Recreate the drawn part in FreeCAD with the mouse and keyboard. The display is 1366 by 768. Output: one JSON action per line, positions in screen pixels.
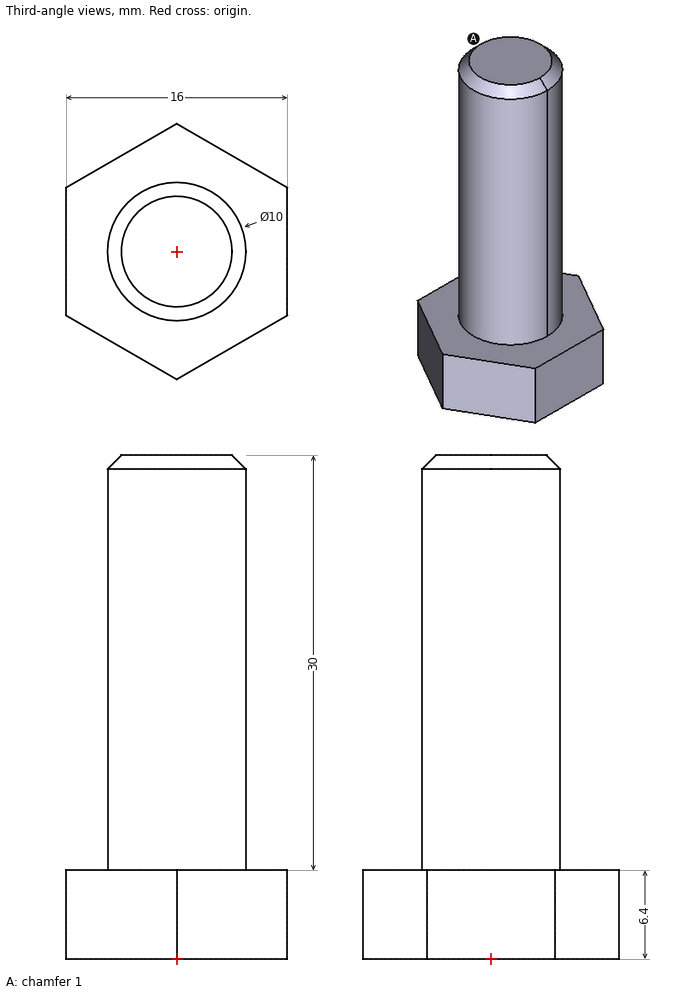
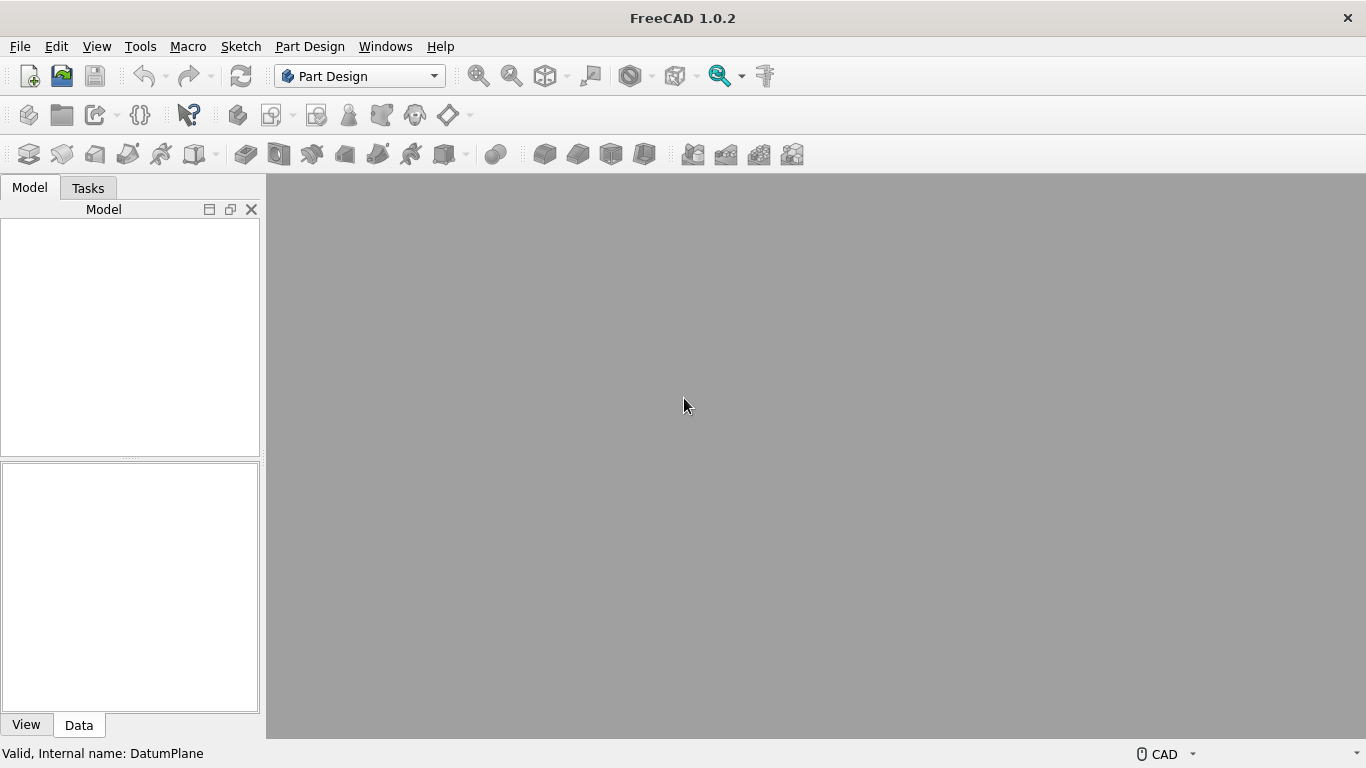
{"action": "left_click", "coordinate": [29, 76]}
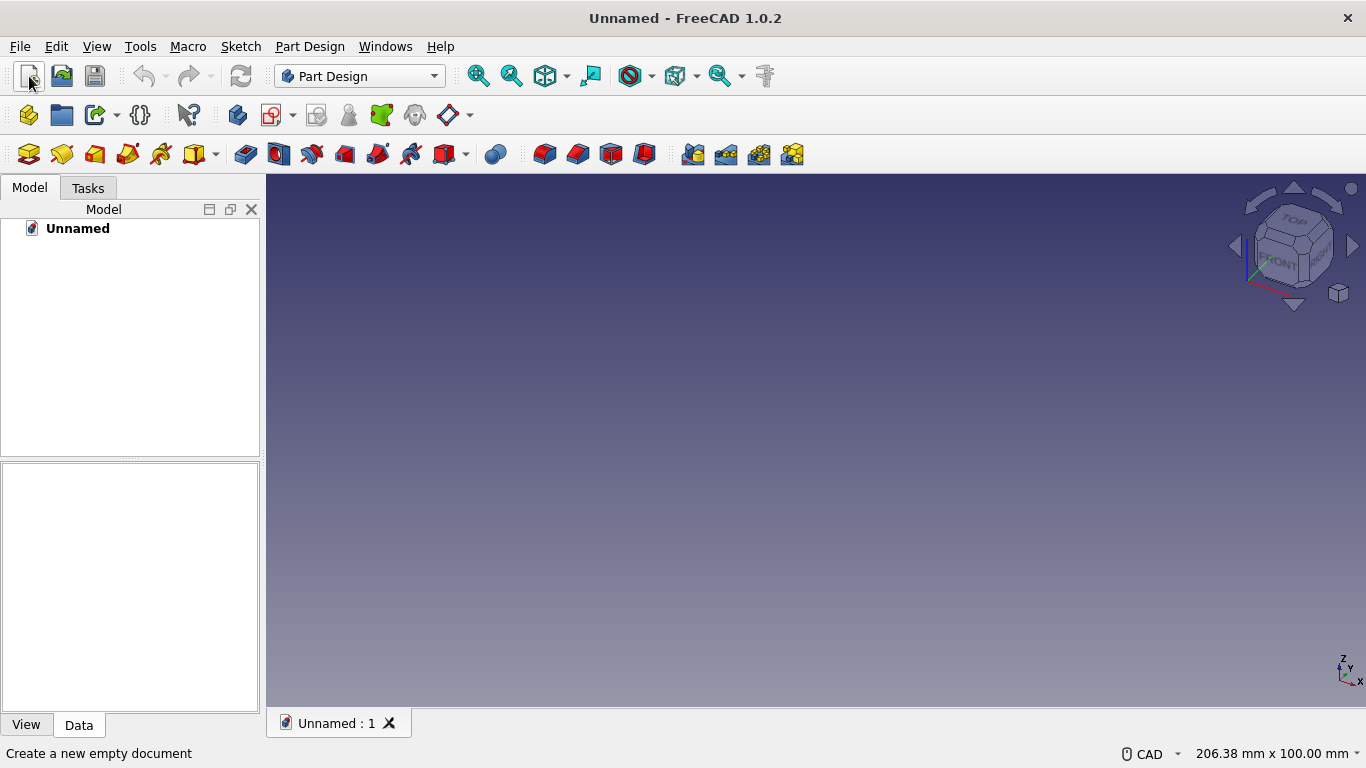
{"action": "left_click", "coordinate": [270, 116]}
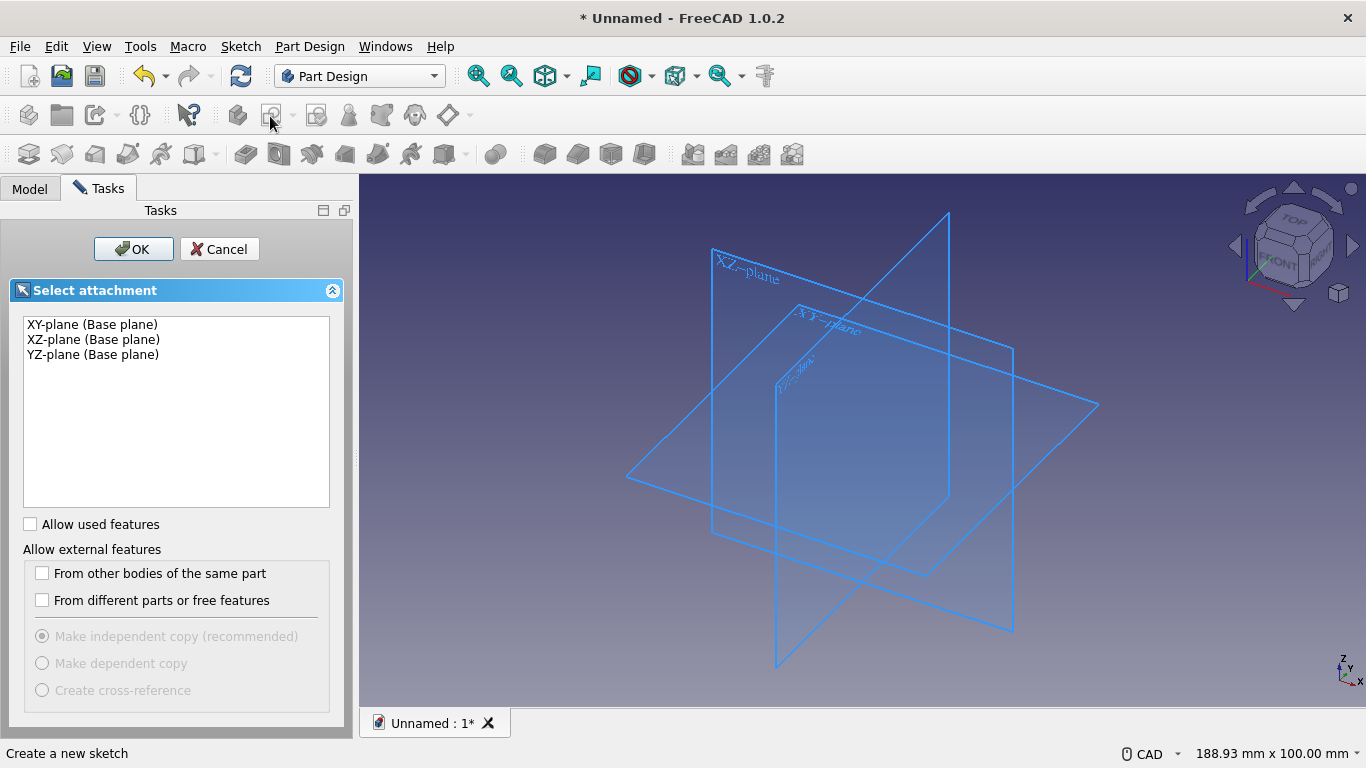
{"action": "left_click", "coordinate": [84, 324]}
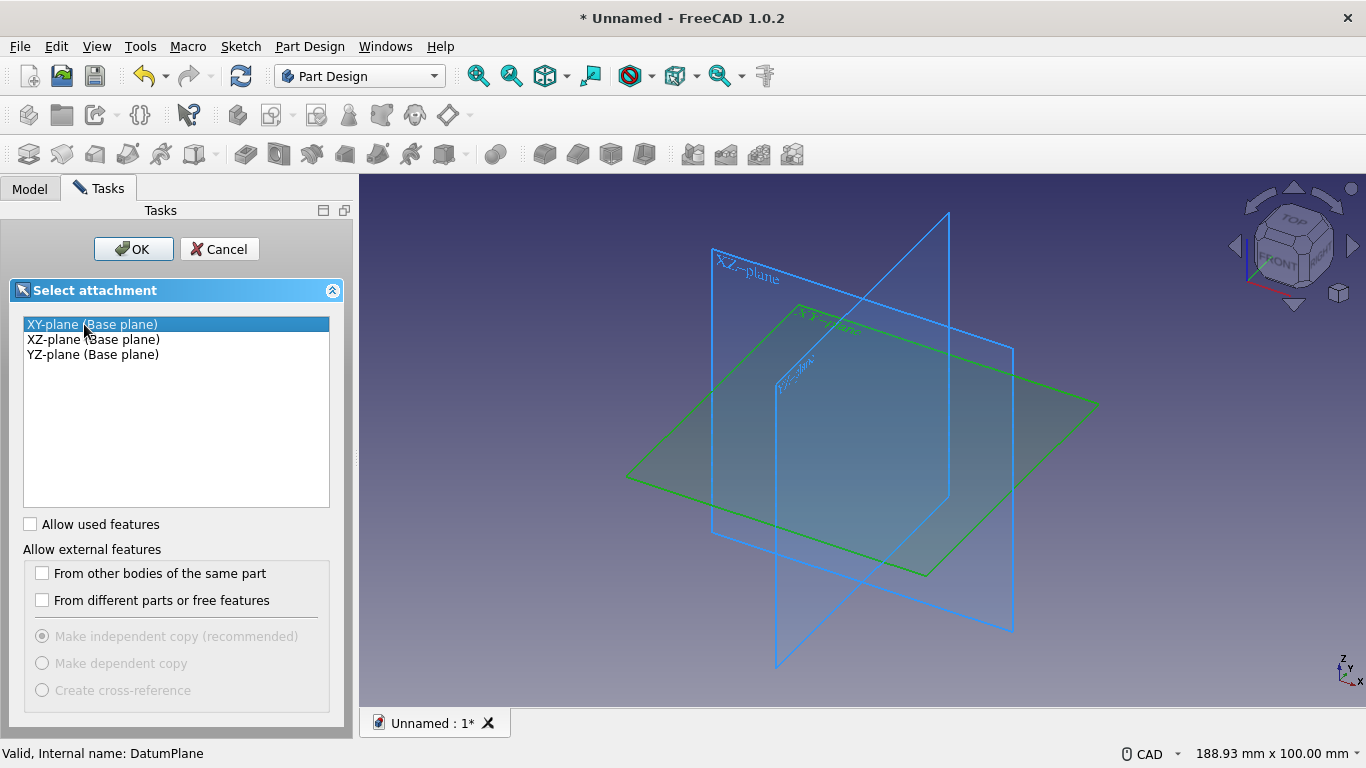
{"action": "left_click", "coordinate": [134, 249]}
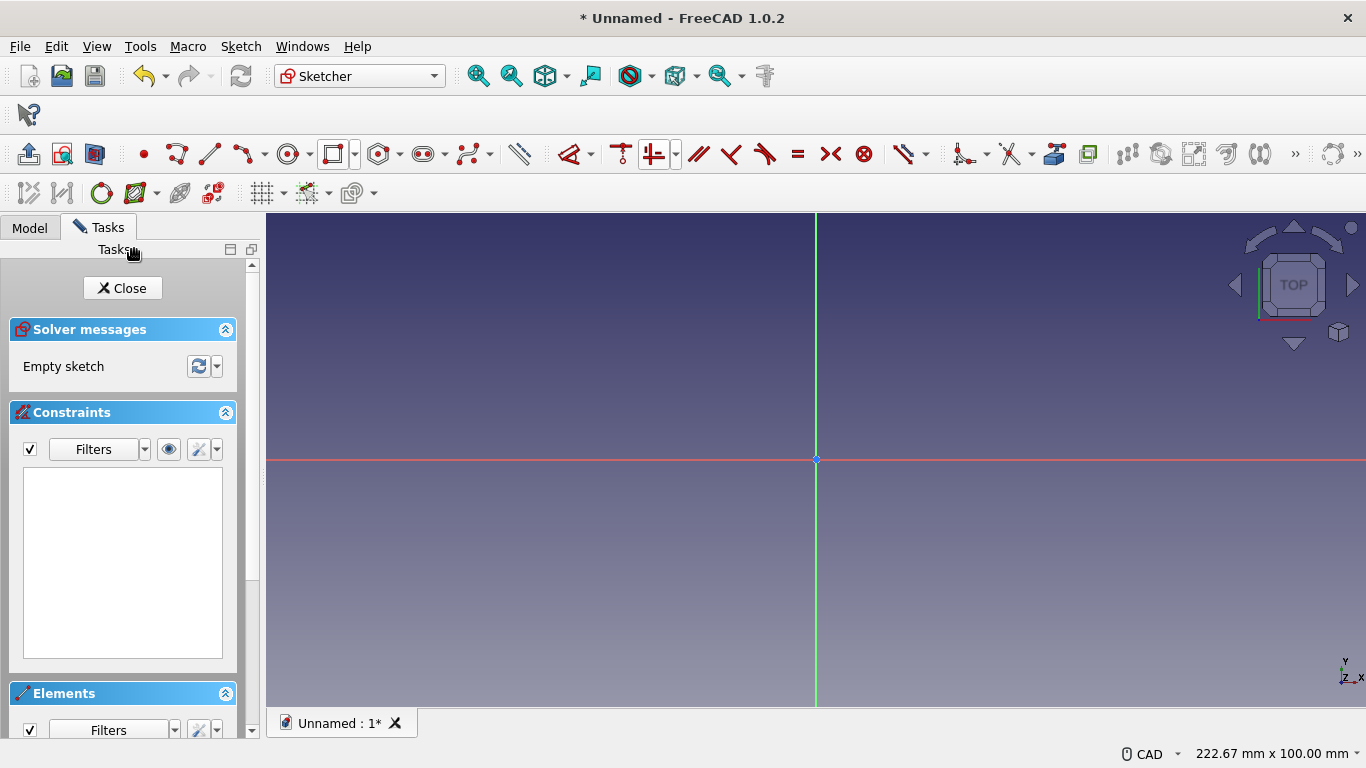
{"action": "scroll", "coordinate": [846, 460], "scroll_direction": "up", "scroll_amount": 6}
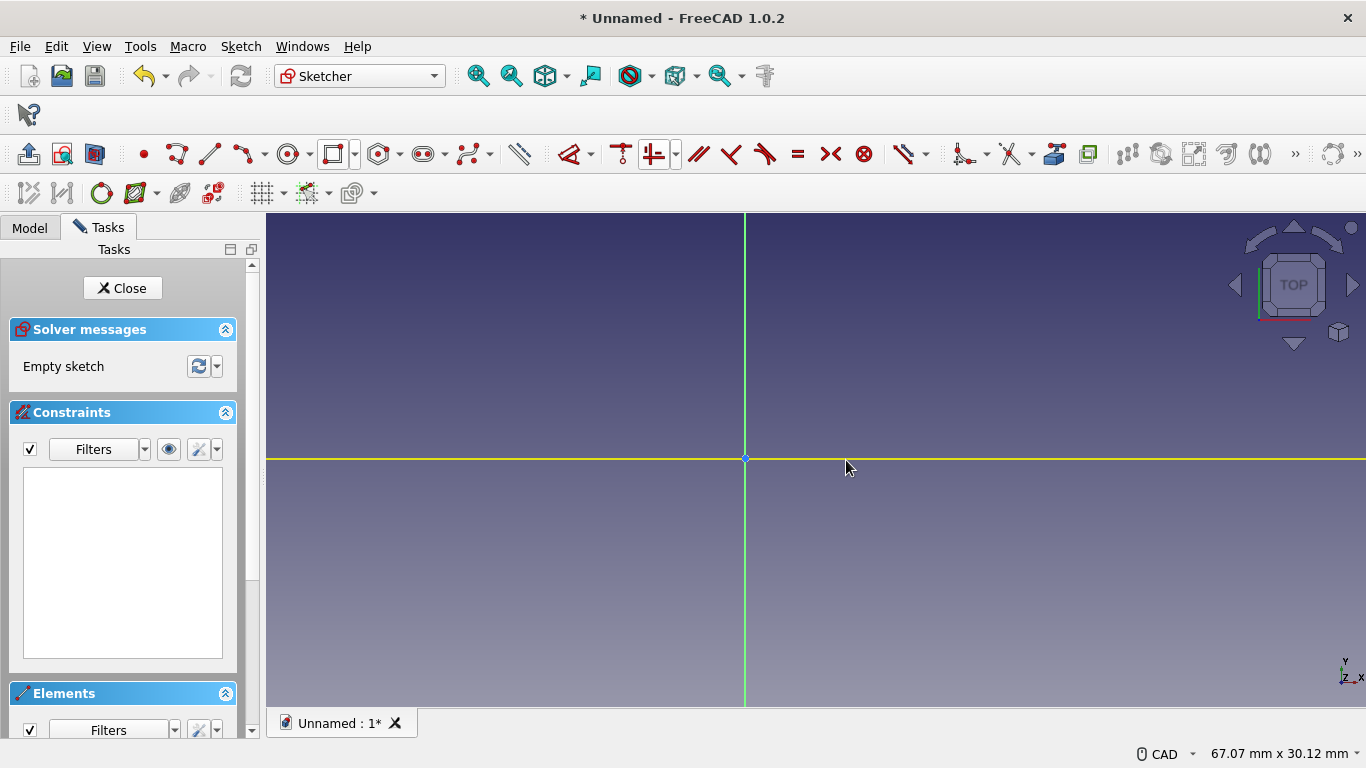
{"action": "key", "text": "g p 6"}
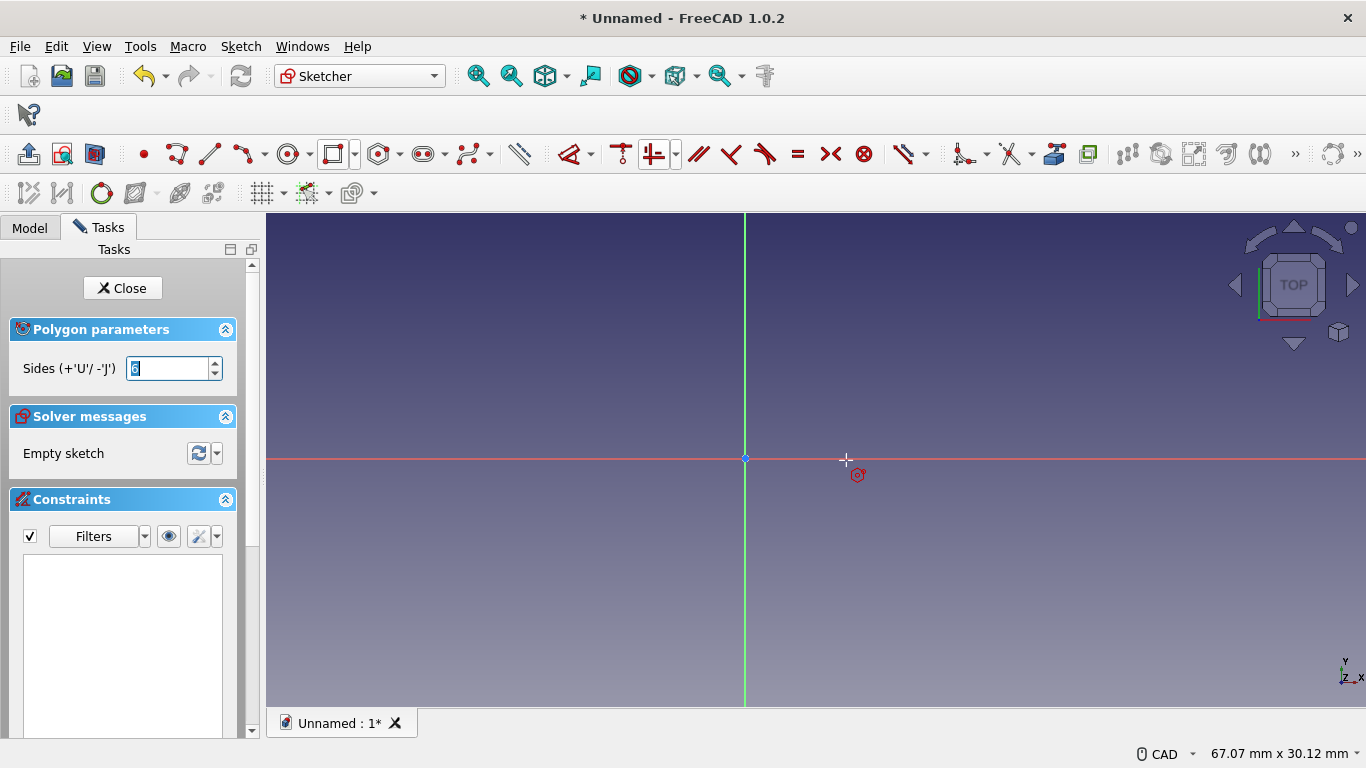
{"action": "left_click", "coordinate": [745, 459]}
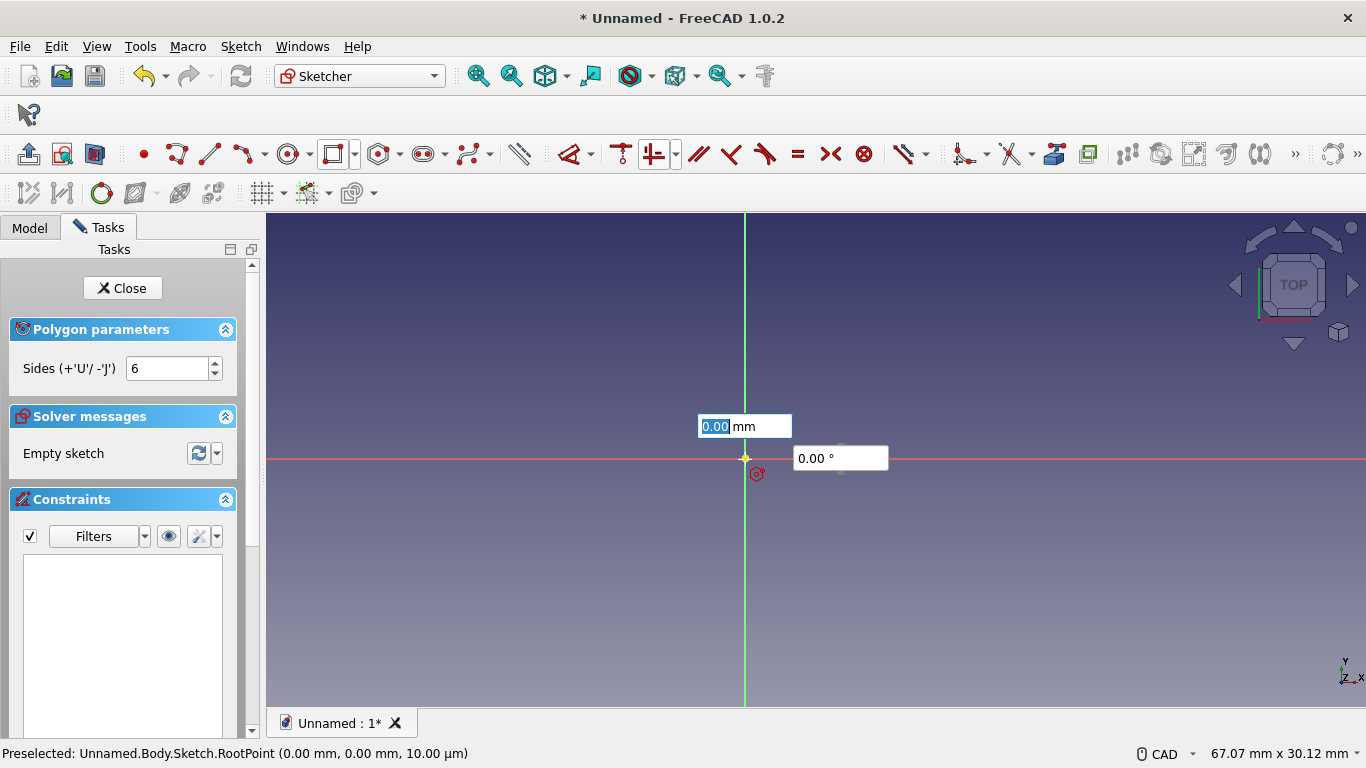
{"action": "left_click", "coordinate": [745, 307]}
{"action": "right_click", "coordinate": [745, 307]}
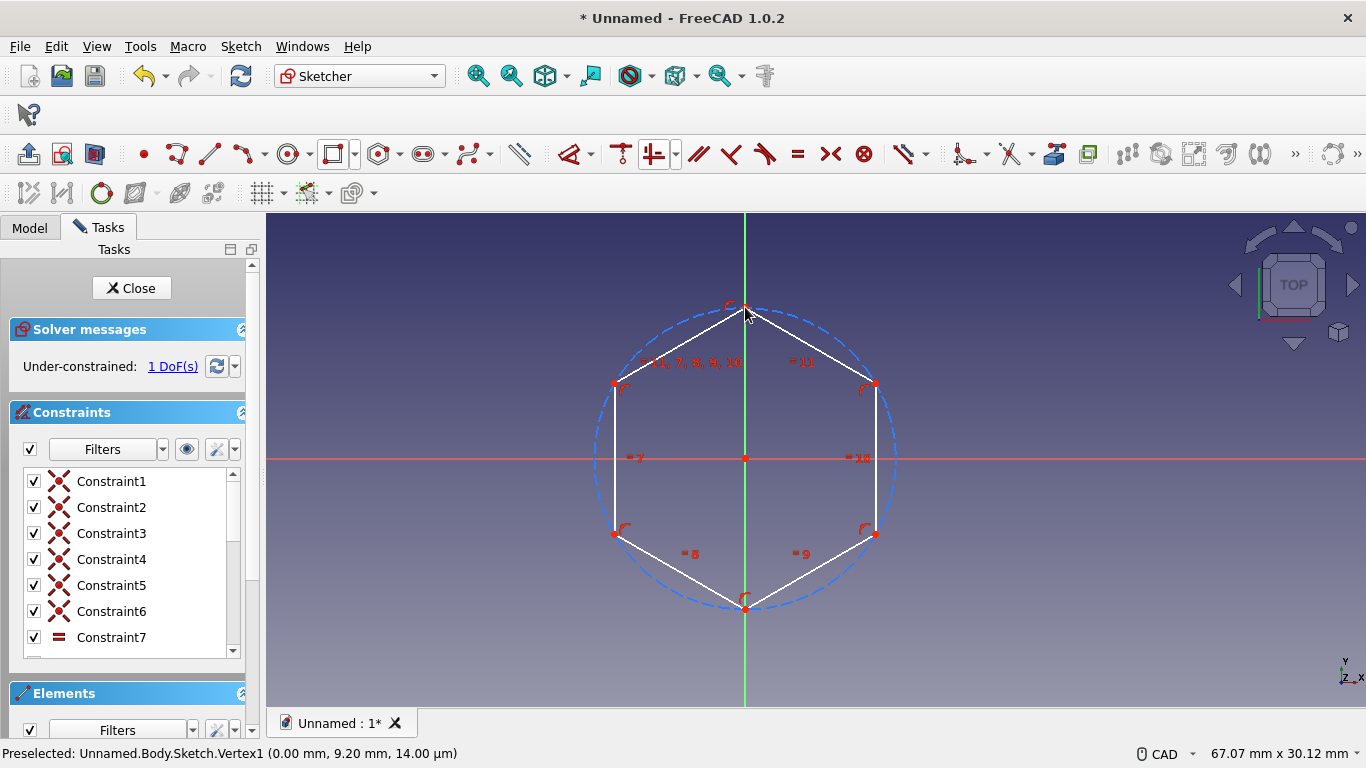
{"action": "left_click", "coordinate": [568, 154]}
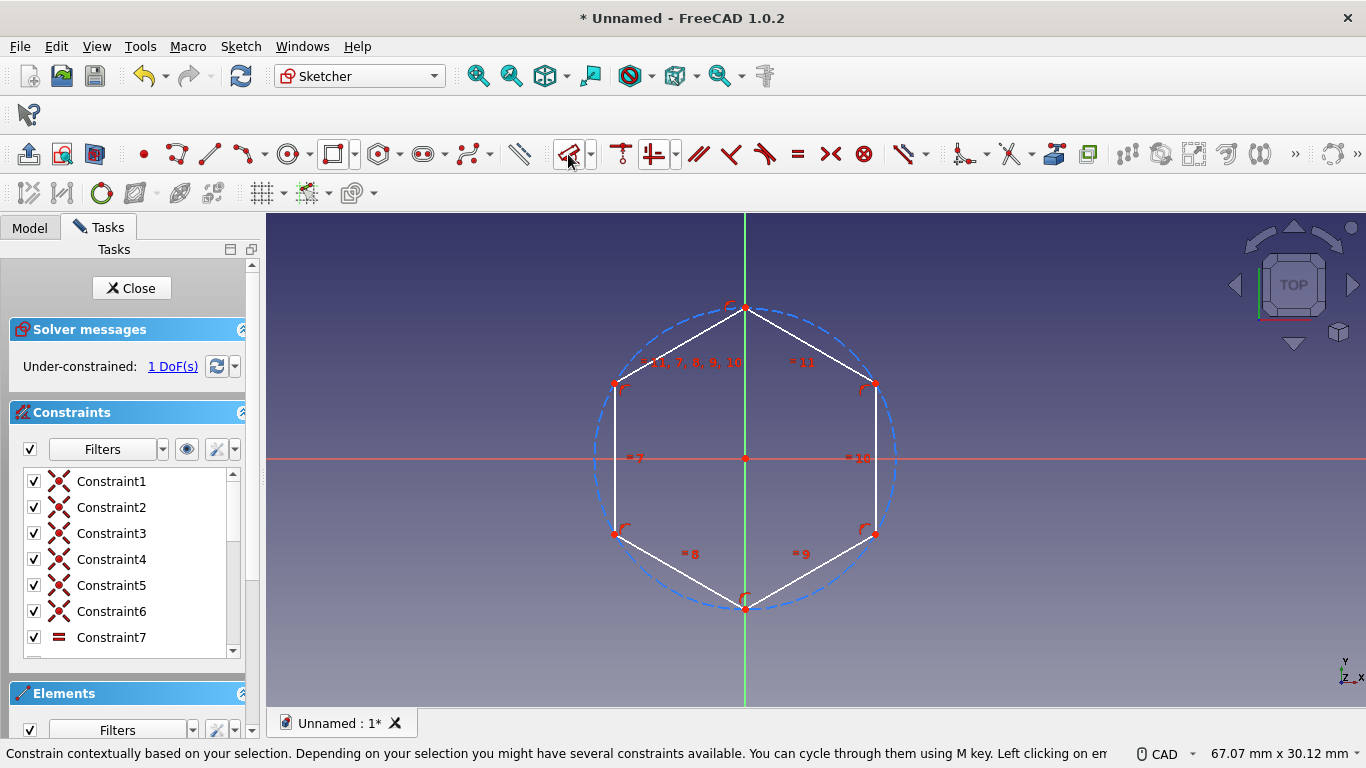
{"action": "left_click", "coordinate": [615, 383]}